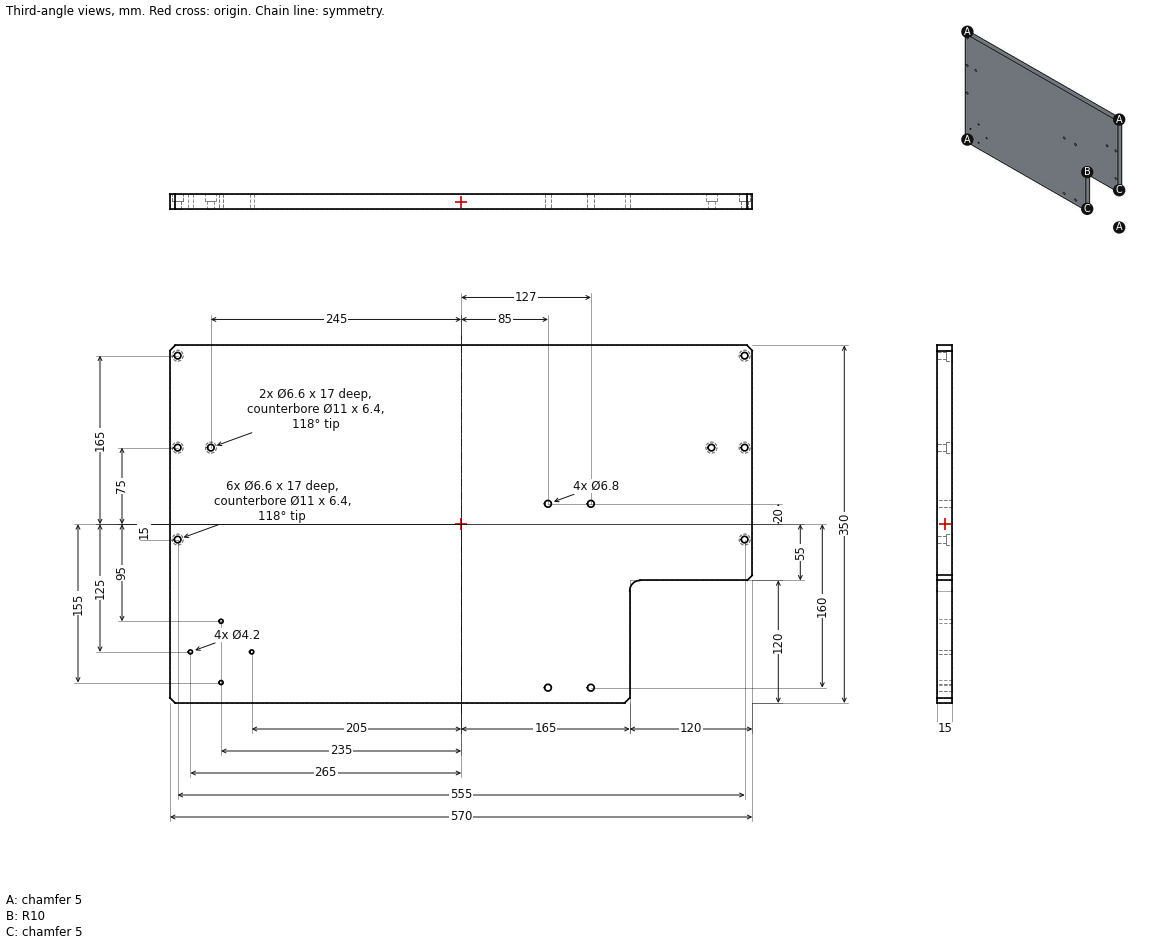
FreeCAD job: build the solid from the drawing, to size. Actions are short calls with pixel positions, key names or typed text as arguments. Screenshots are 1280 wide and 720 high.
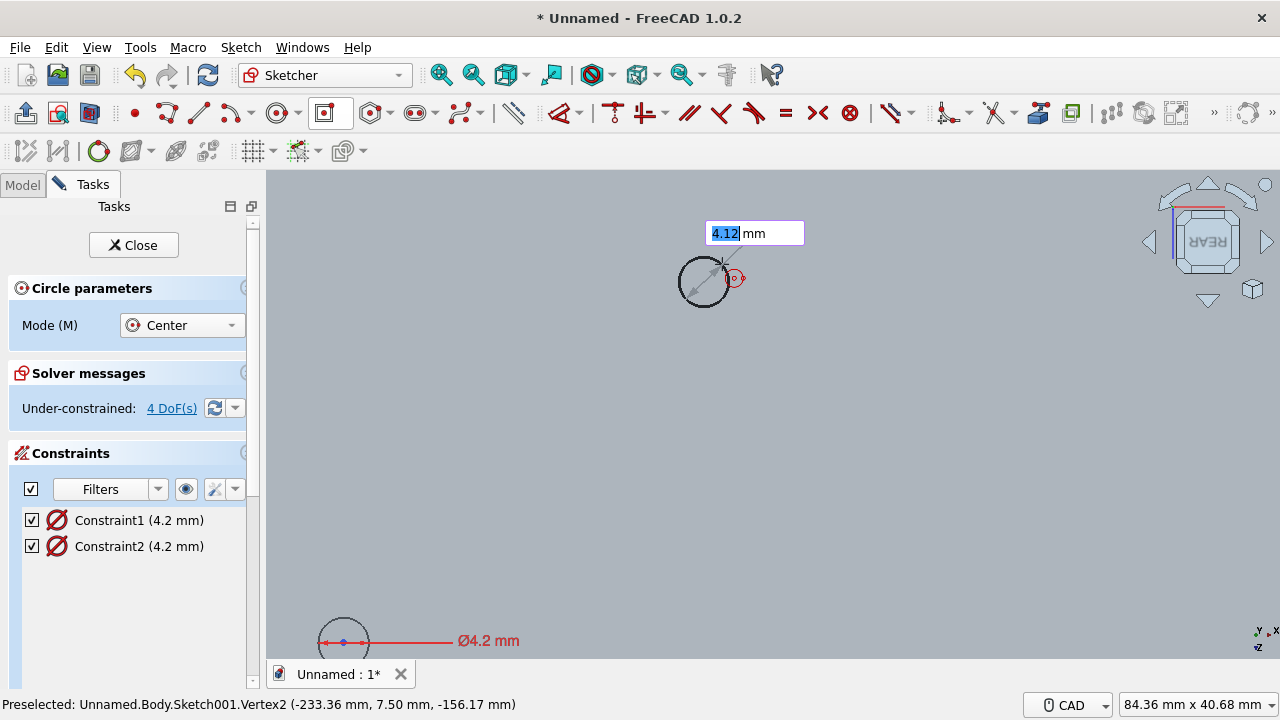
text(4.2)
key(Return)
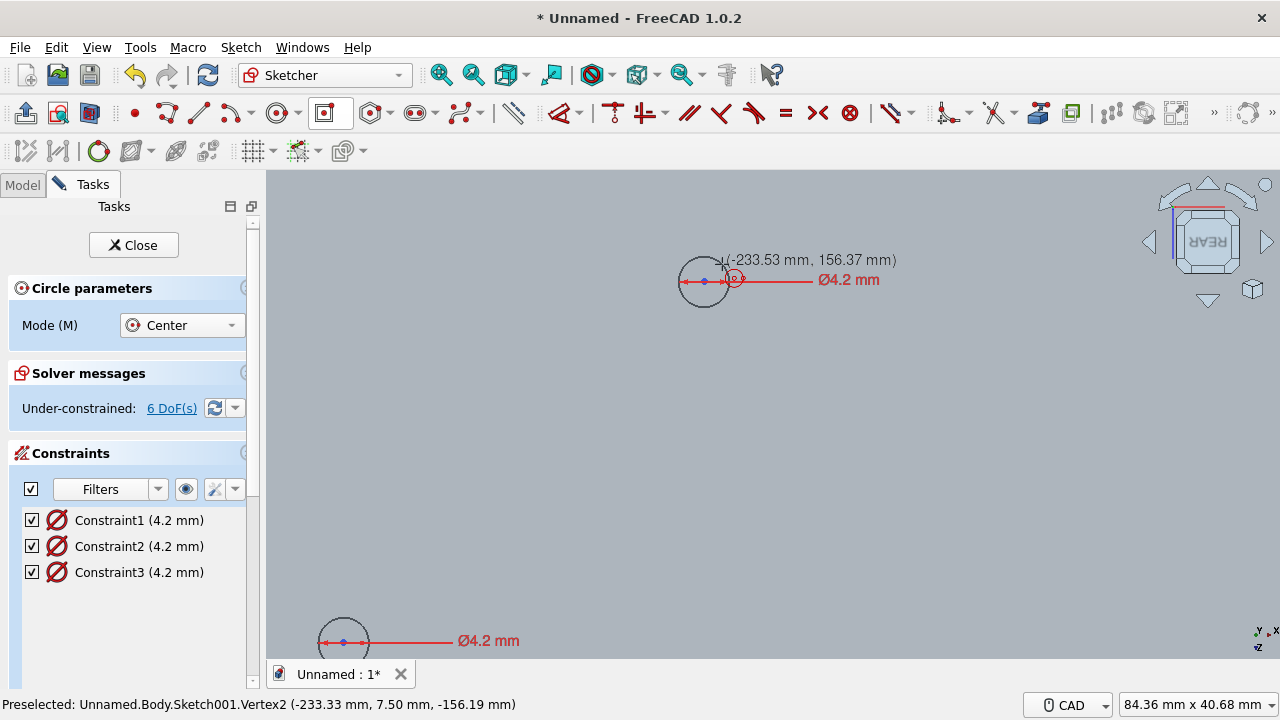
scroll(705, 282, down, 5)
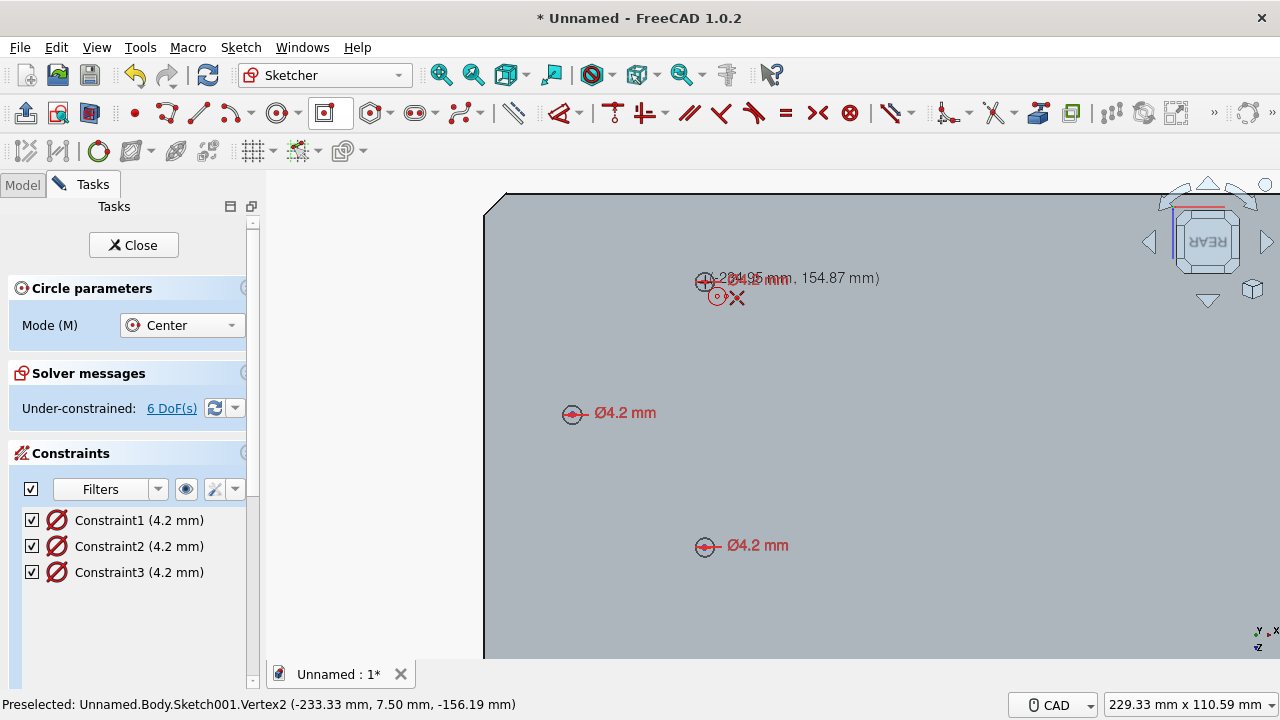
scroll(838, 415, up, 5)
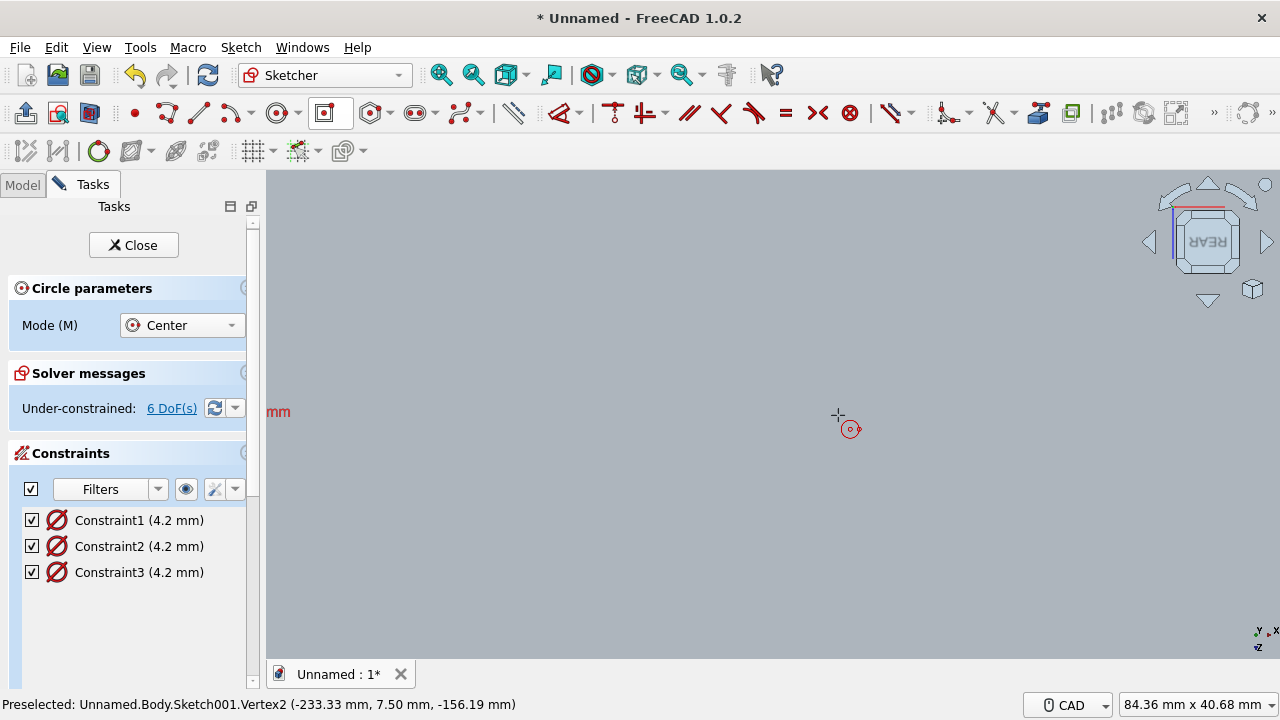
click(836, 413)
move(854, 395)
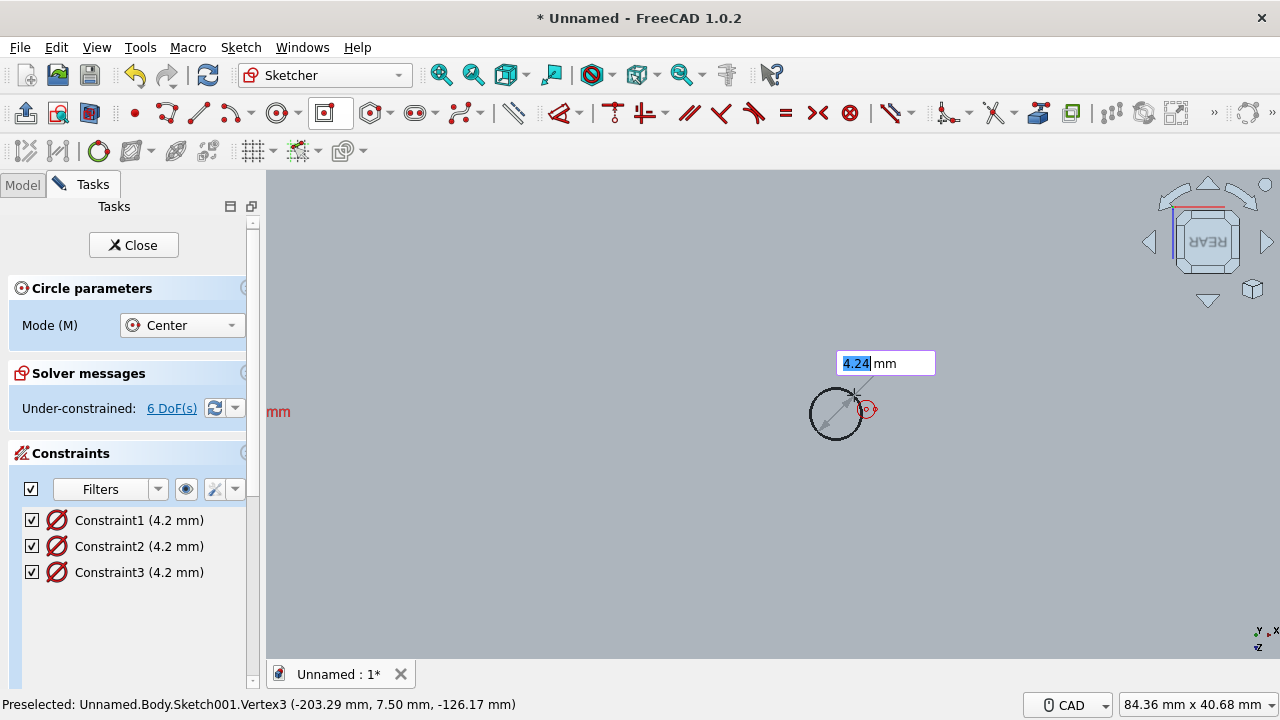
text(4.2)
key(Return)
key(Escape)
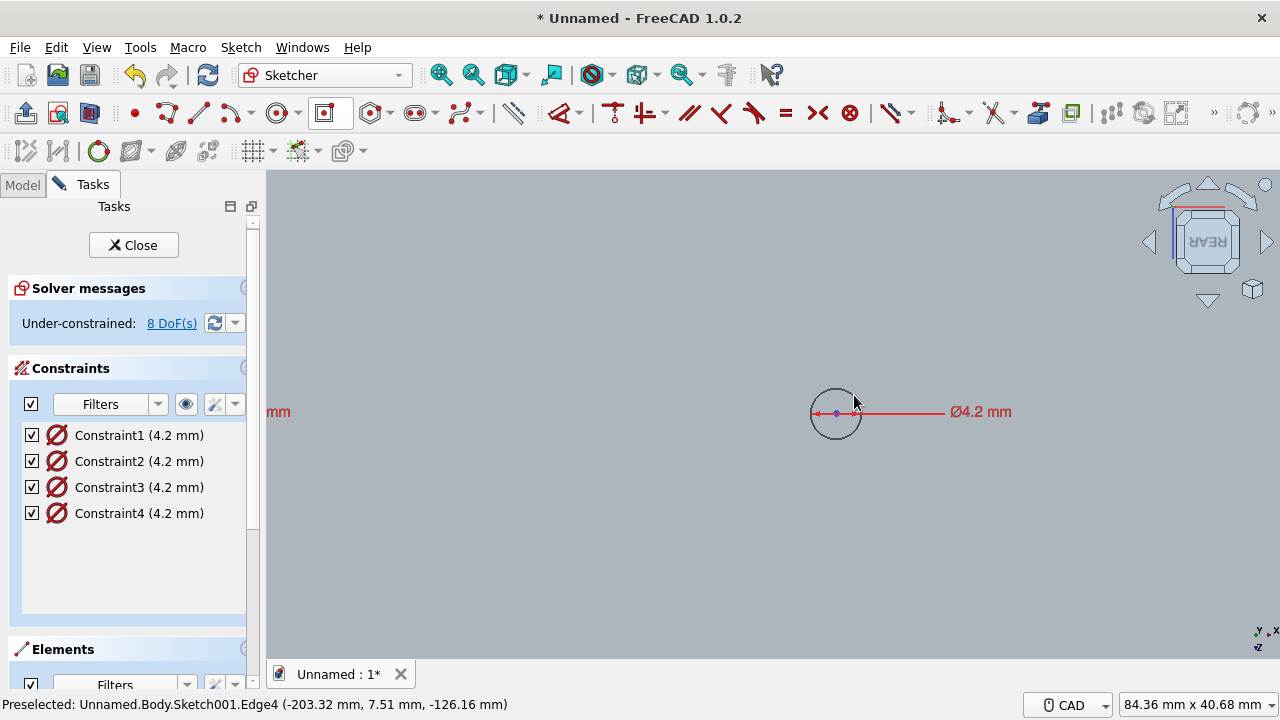
click(560, 114)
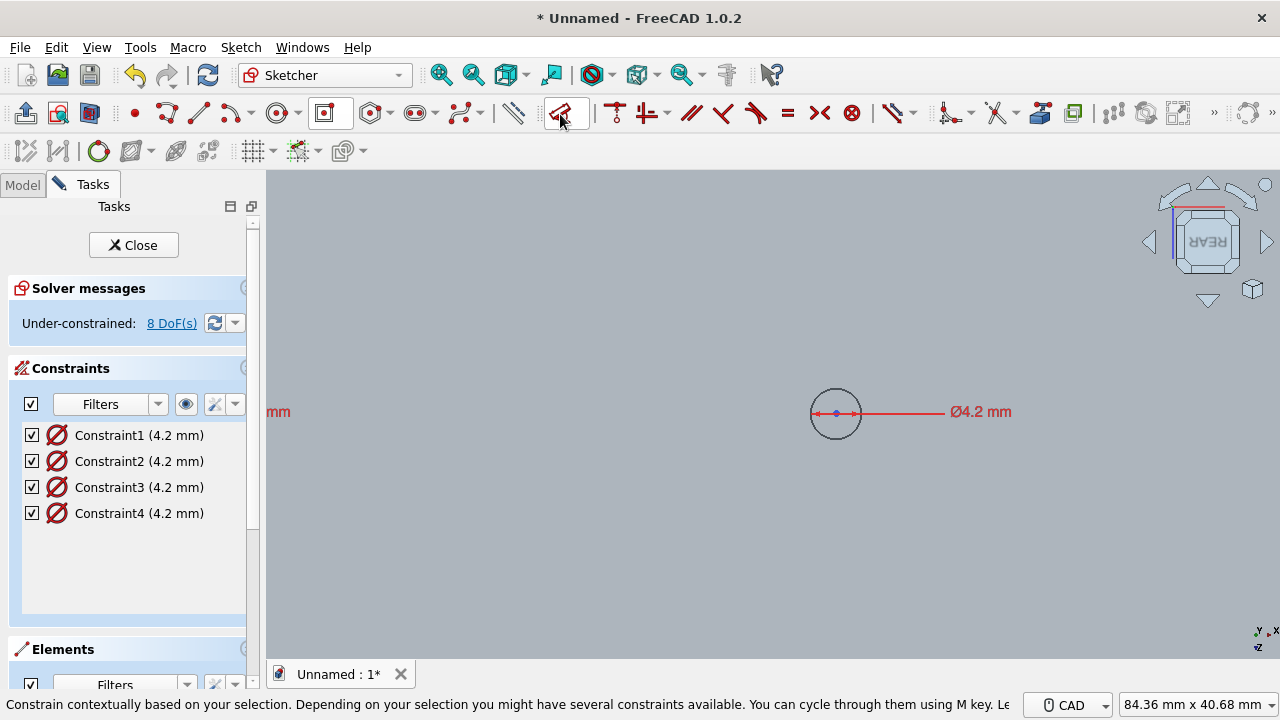
scroll(838, 415, down, 5)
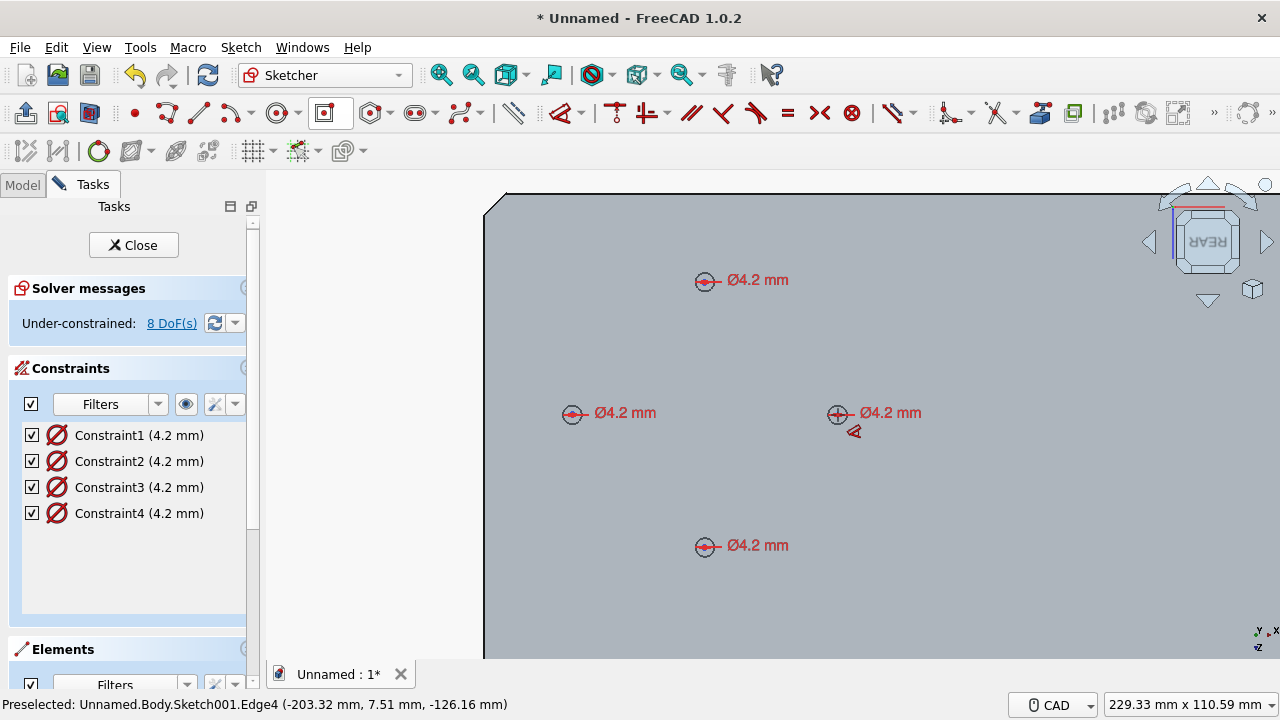
click(705, 547)
click(671, 589)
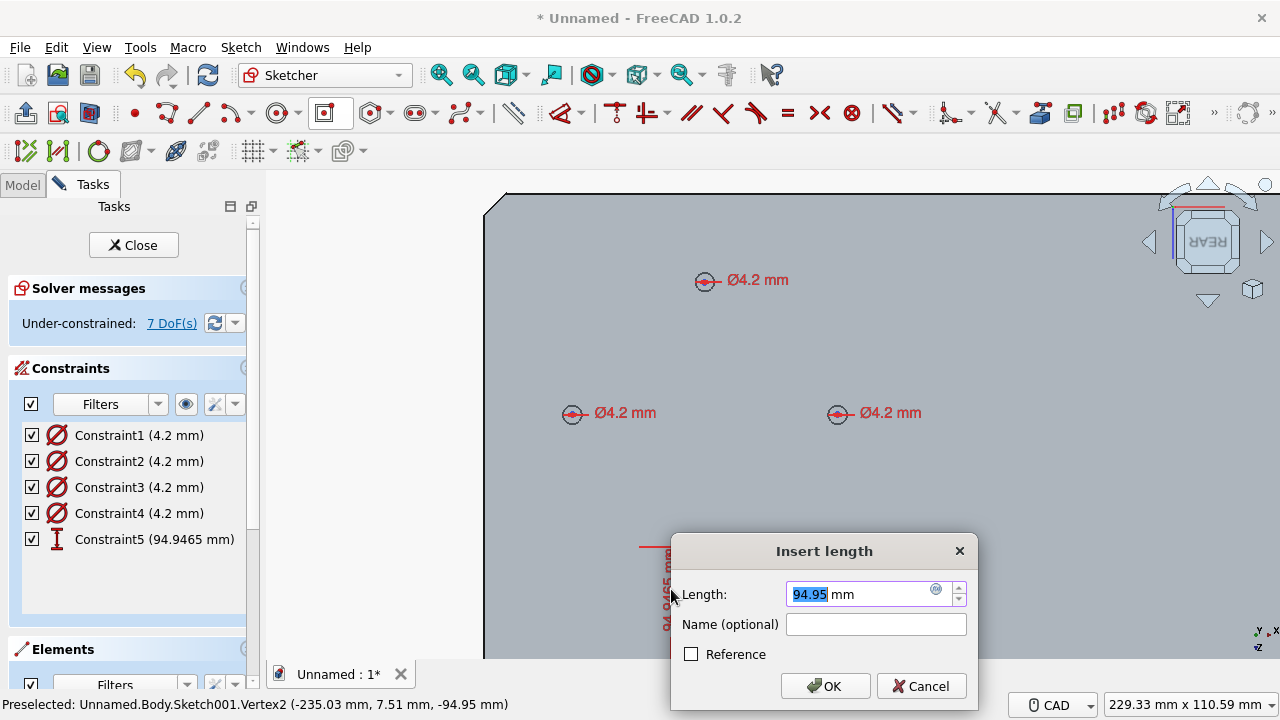
text(95)
key(Return)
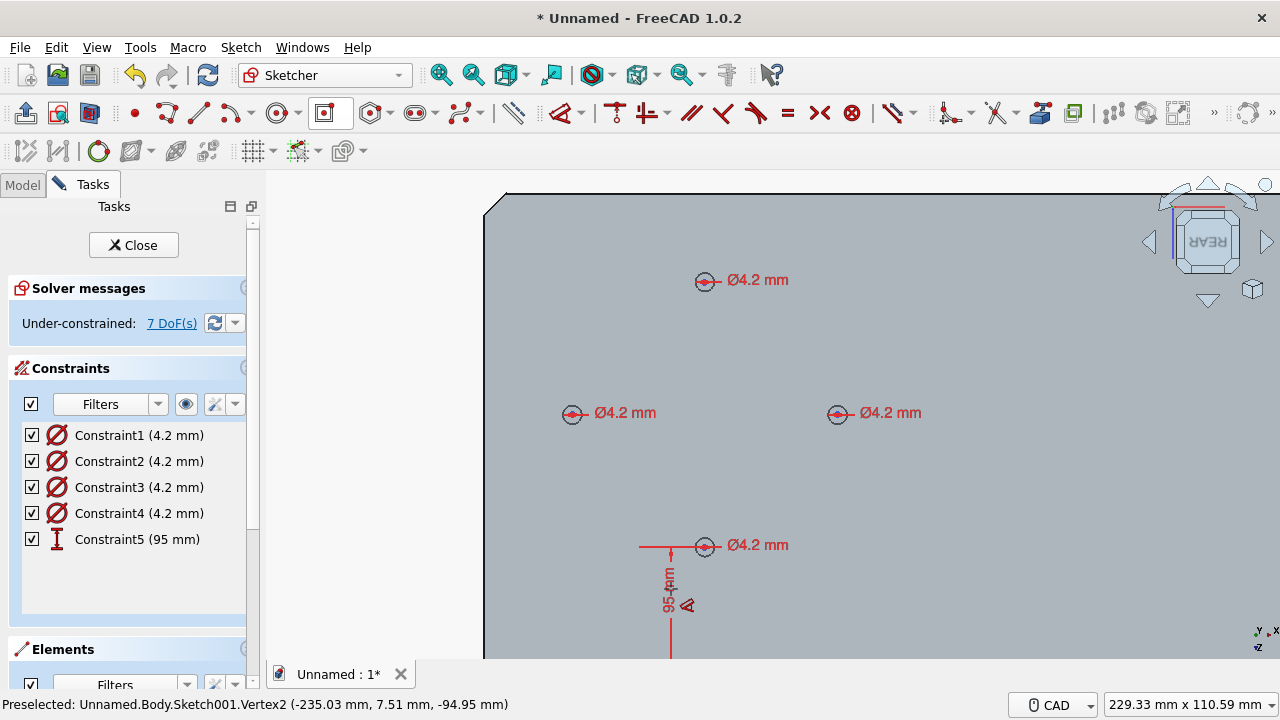
click(572, 415)
click(844, 381)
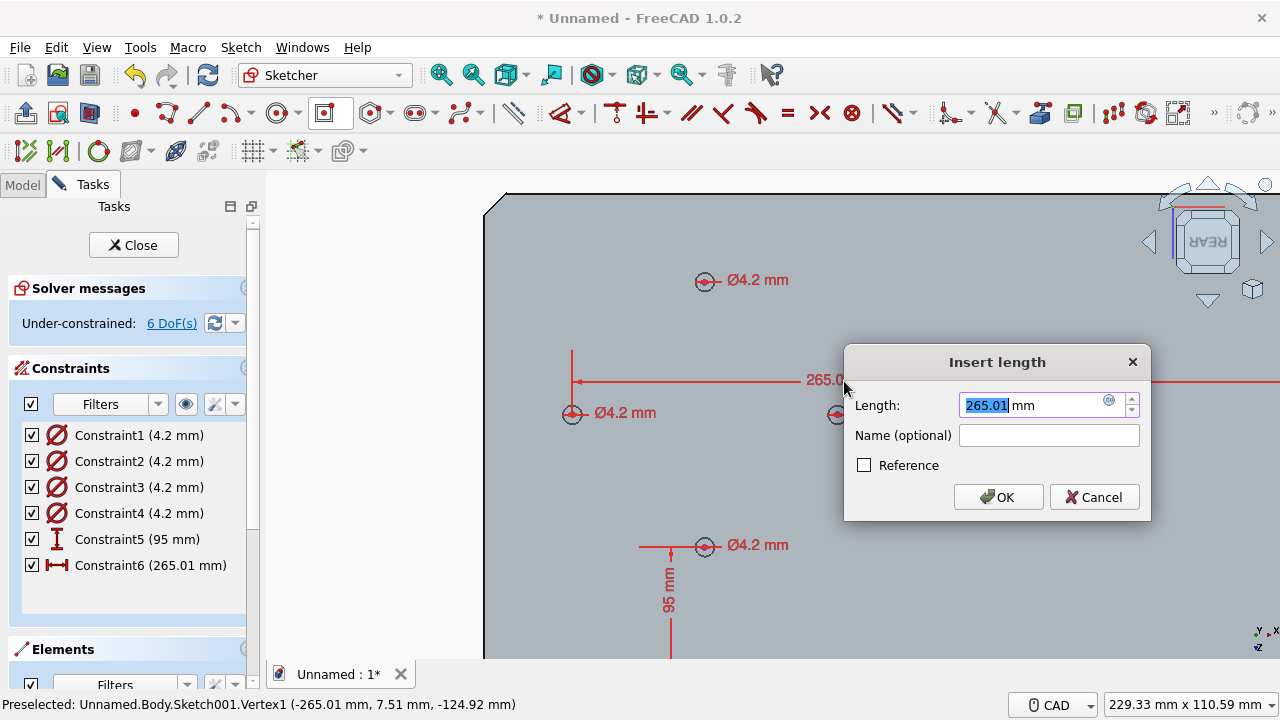
text(265)
key(Return)